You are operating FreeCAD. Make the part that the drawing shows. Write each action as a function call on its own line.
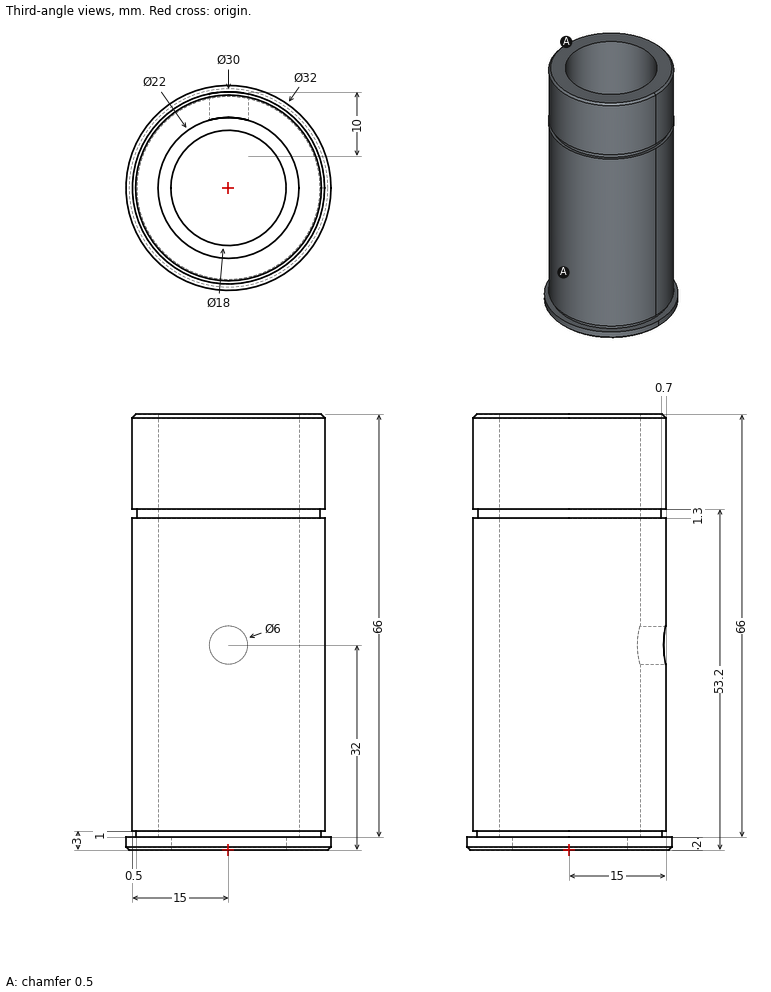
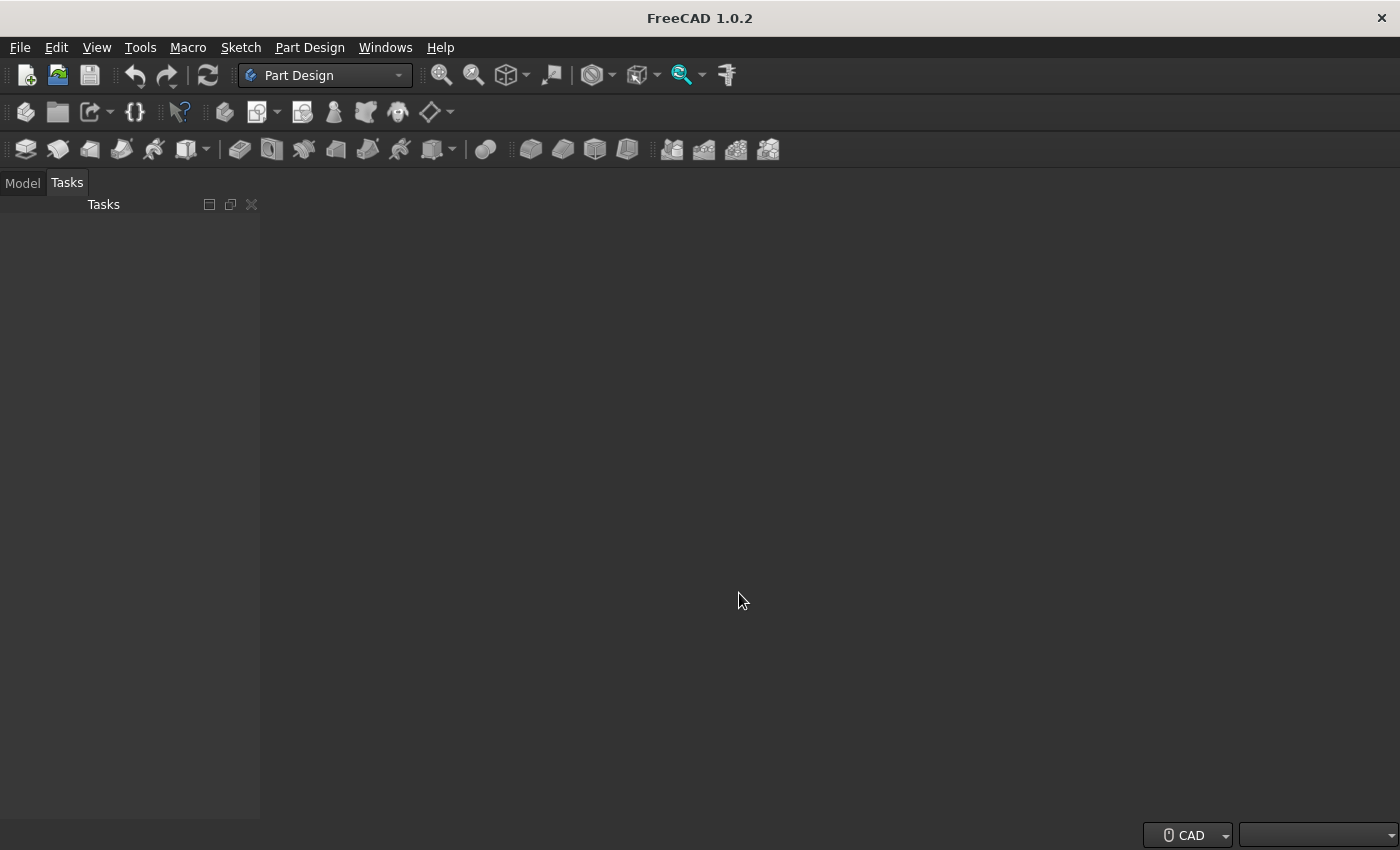
click(26, 76)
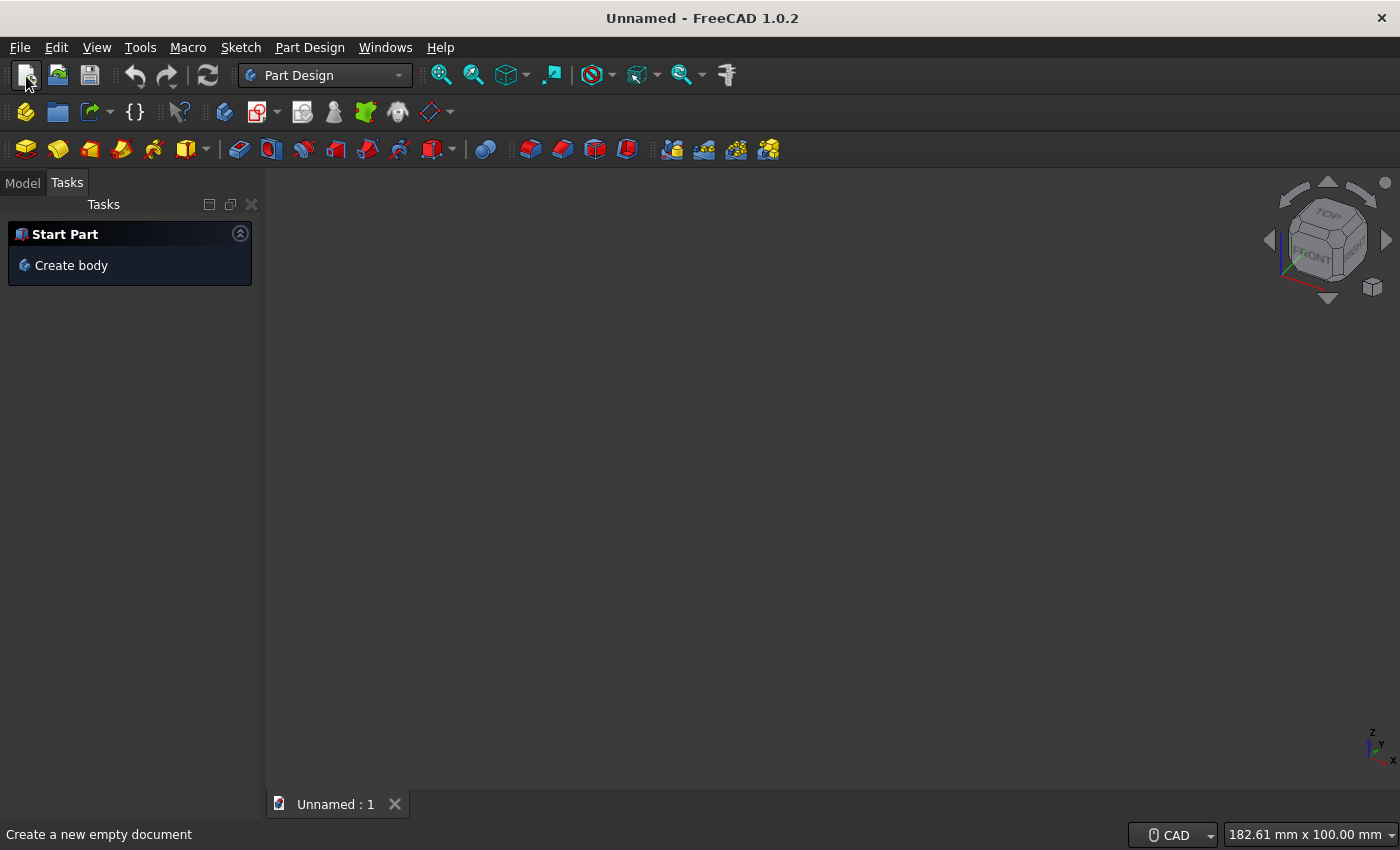
click(258, 112)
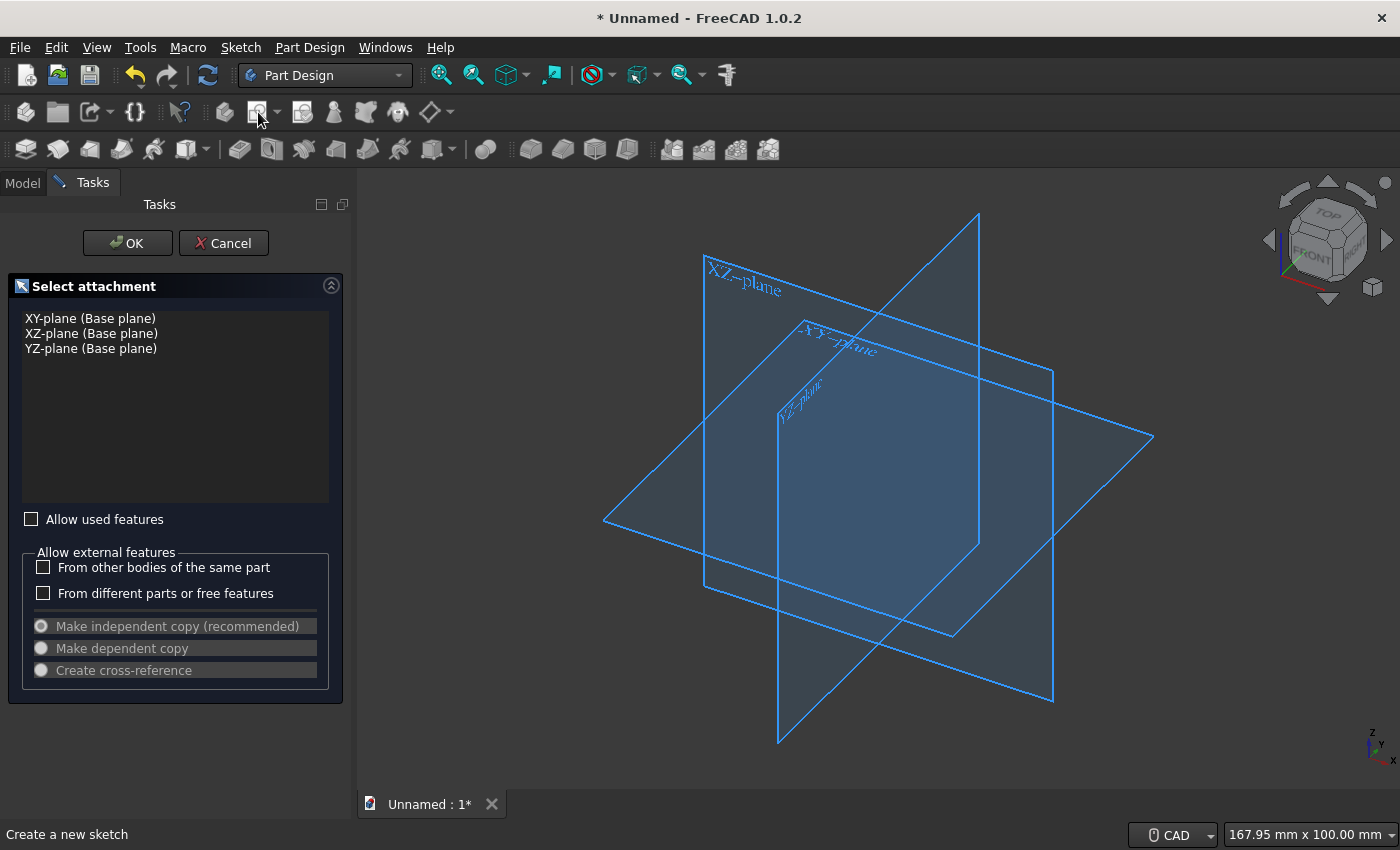
click(82, 318)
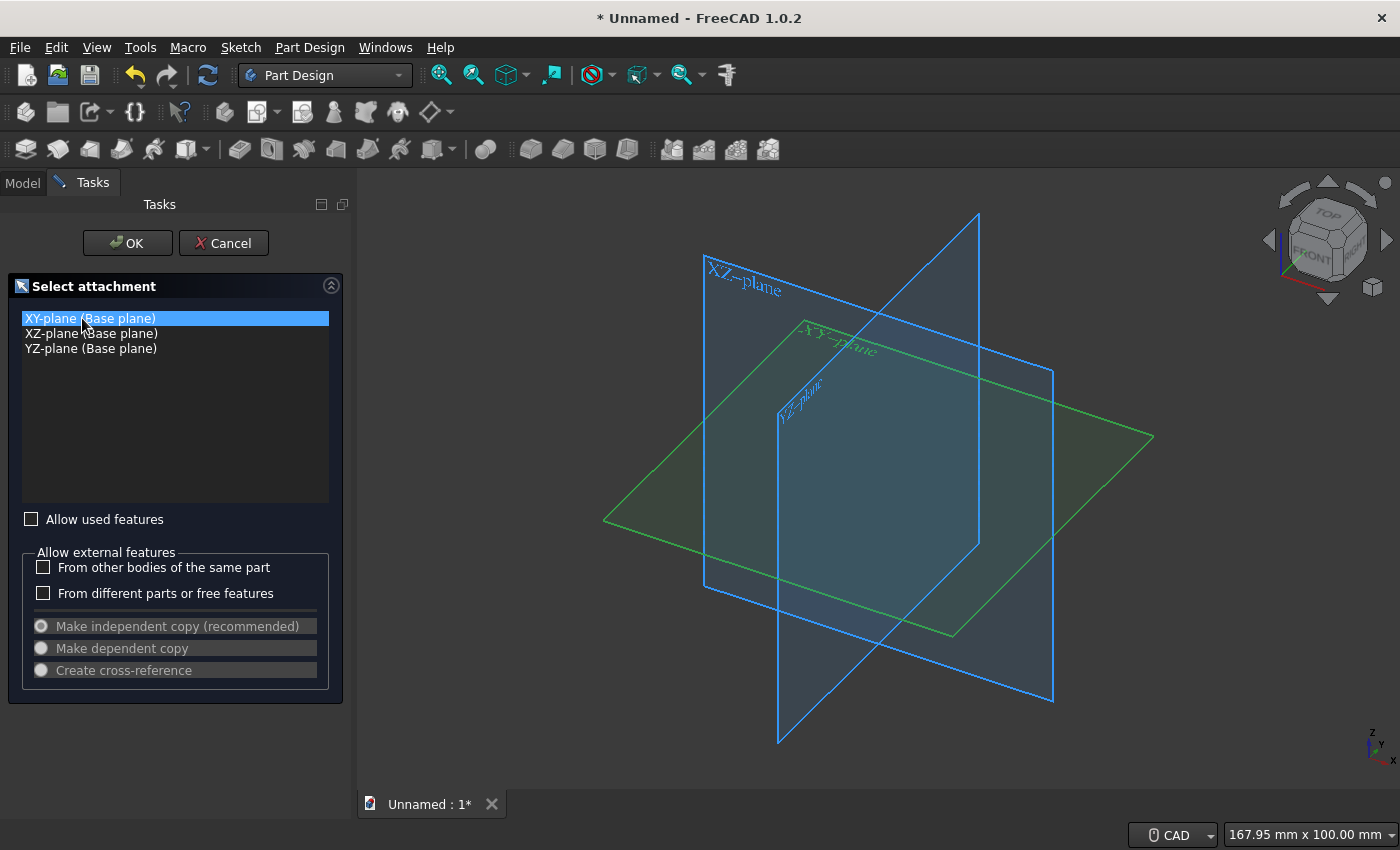
click(128, 243)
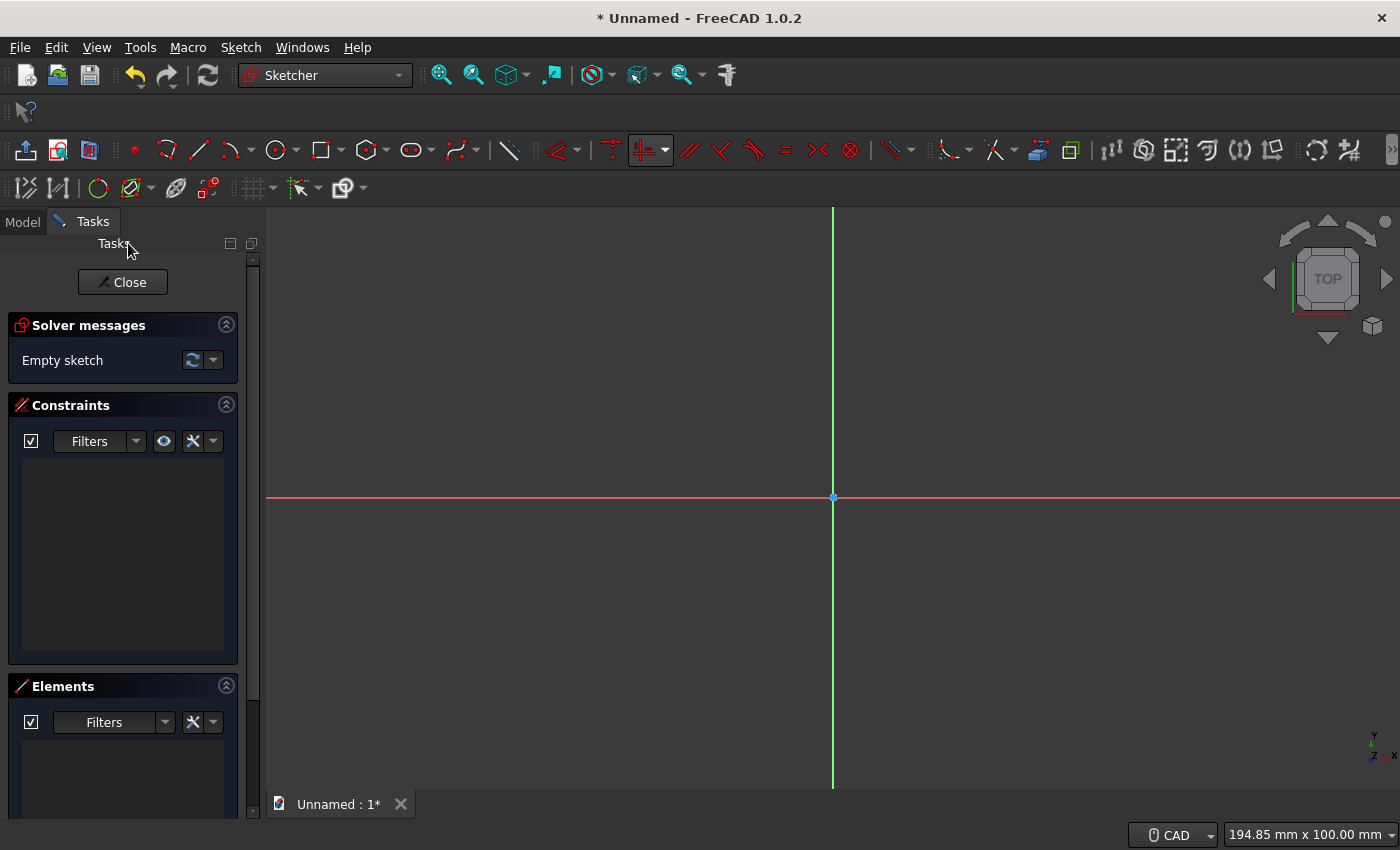
scroll(916, 498, up, 3)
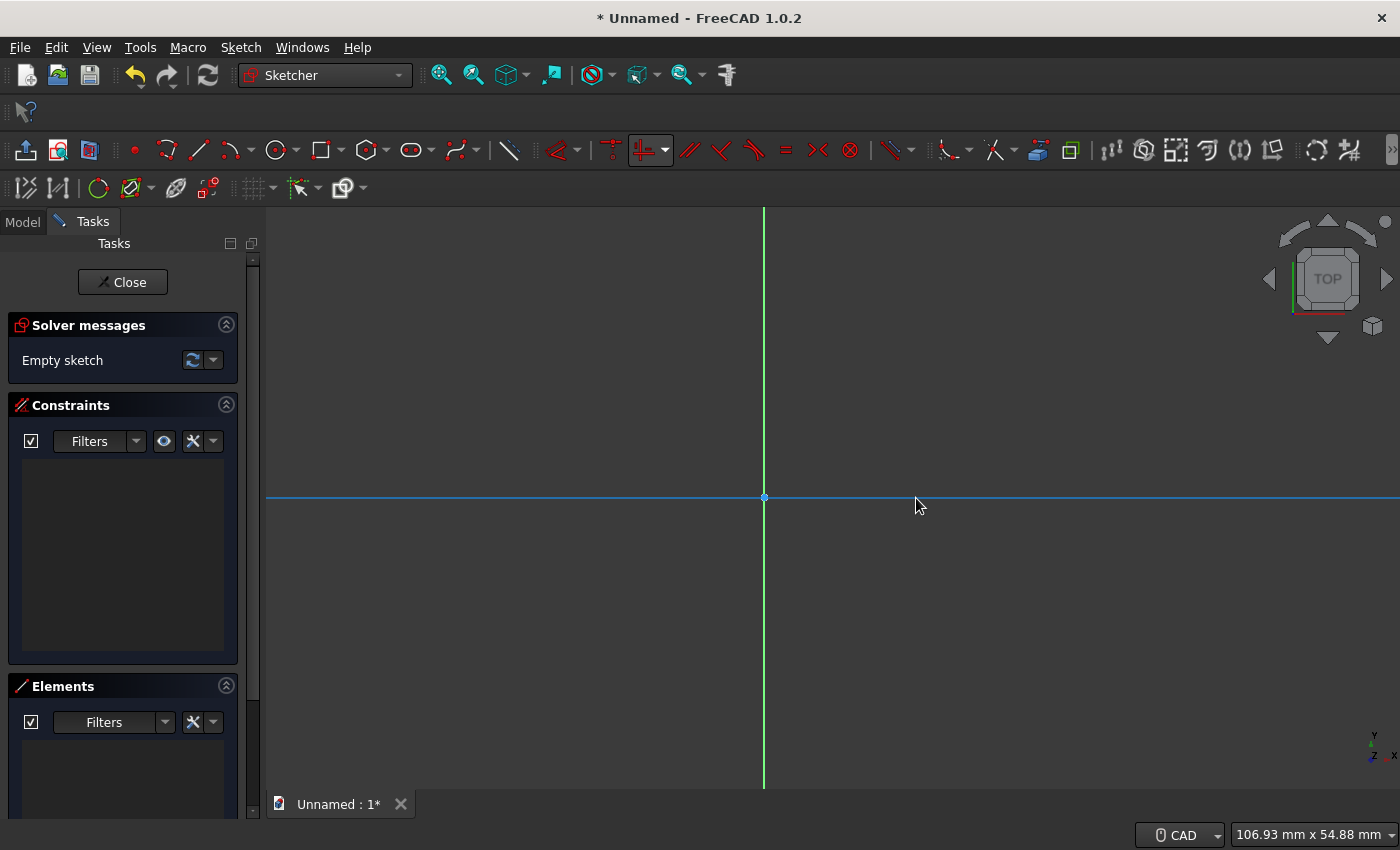
key(g)
key(c)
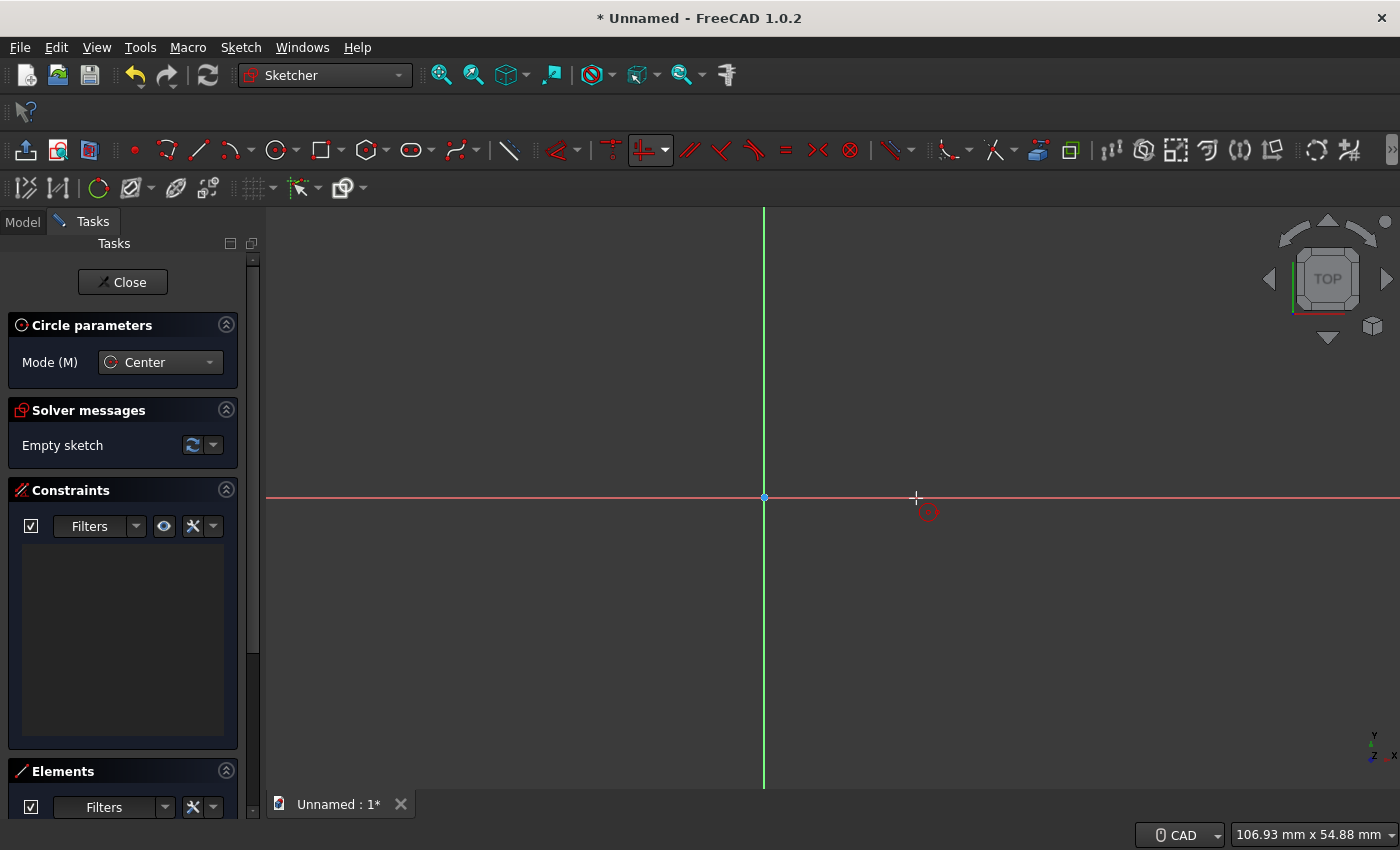
click(764, 498)
move(884, 378)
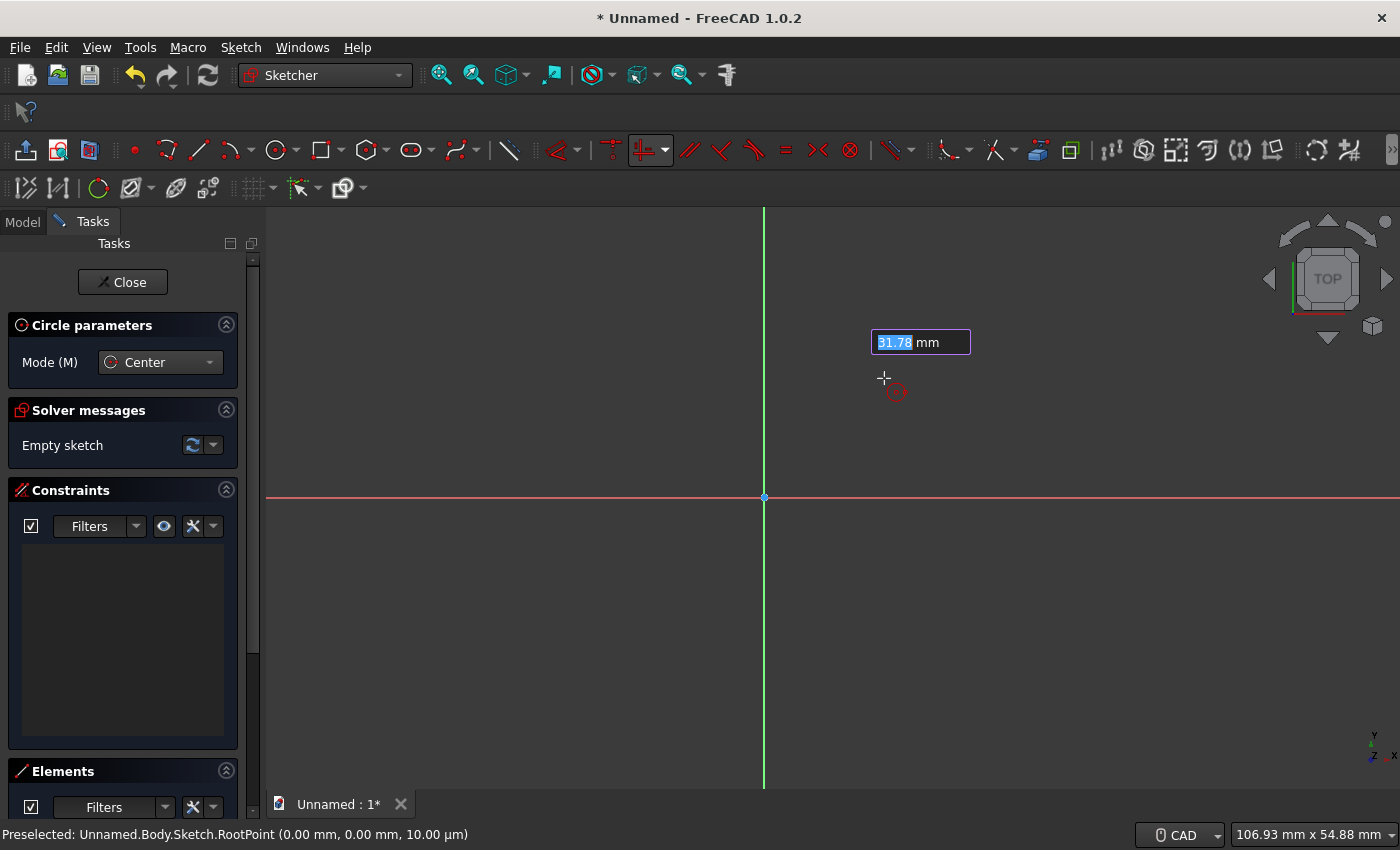
text(32)
key(Return)
key(Escape)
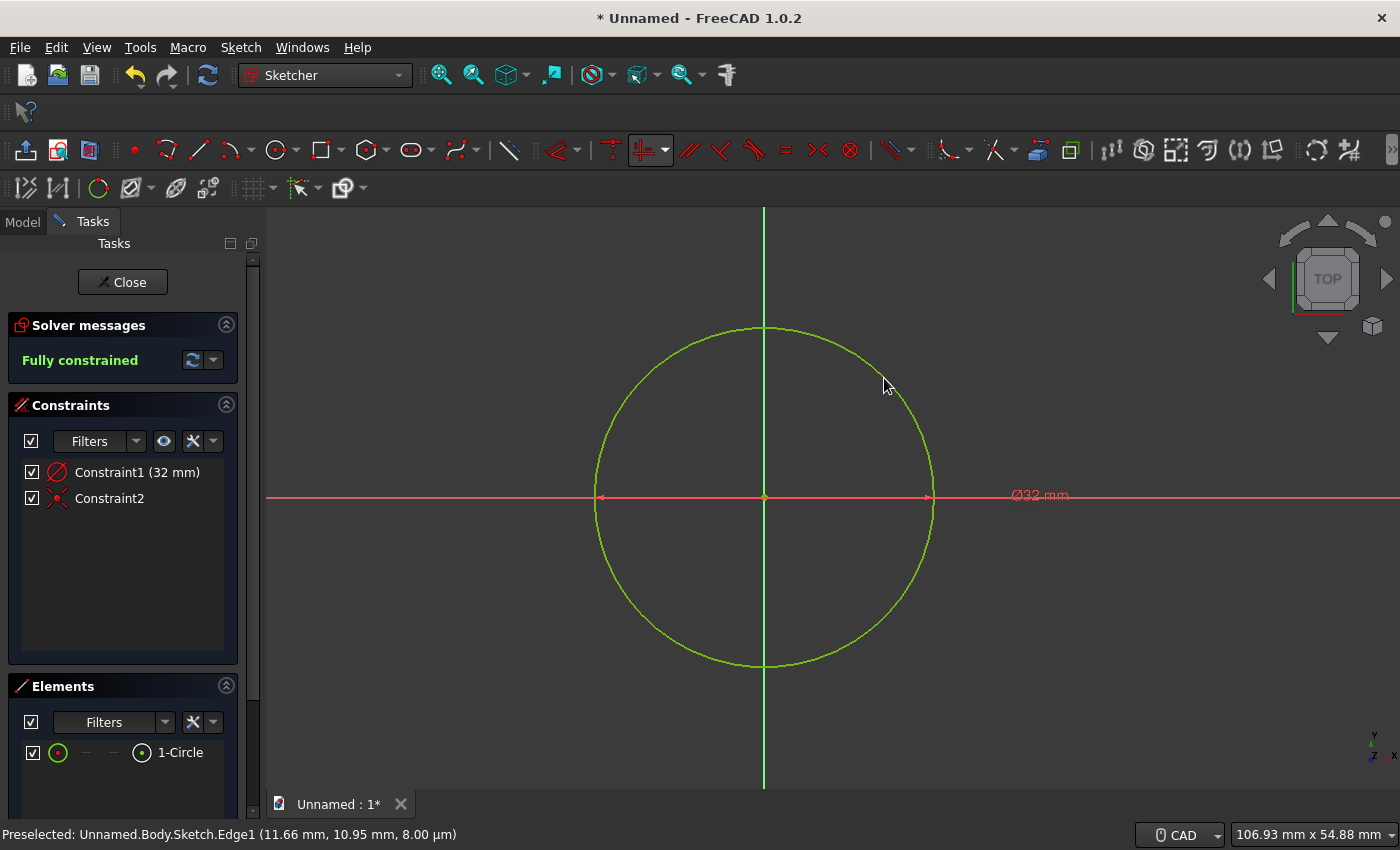
click(123, 282)